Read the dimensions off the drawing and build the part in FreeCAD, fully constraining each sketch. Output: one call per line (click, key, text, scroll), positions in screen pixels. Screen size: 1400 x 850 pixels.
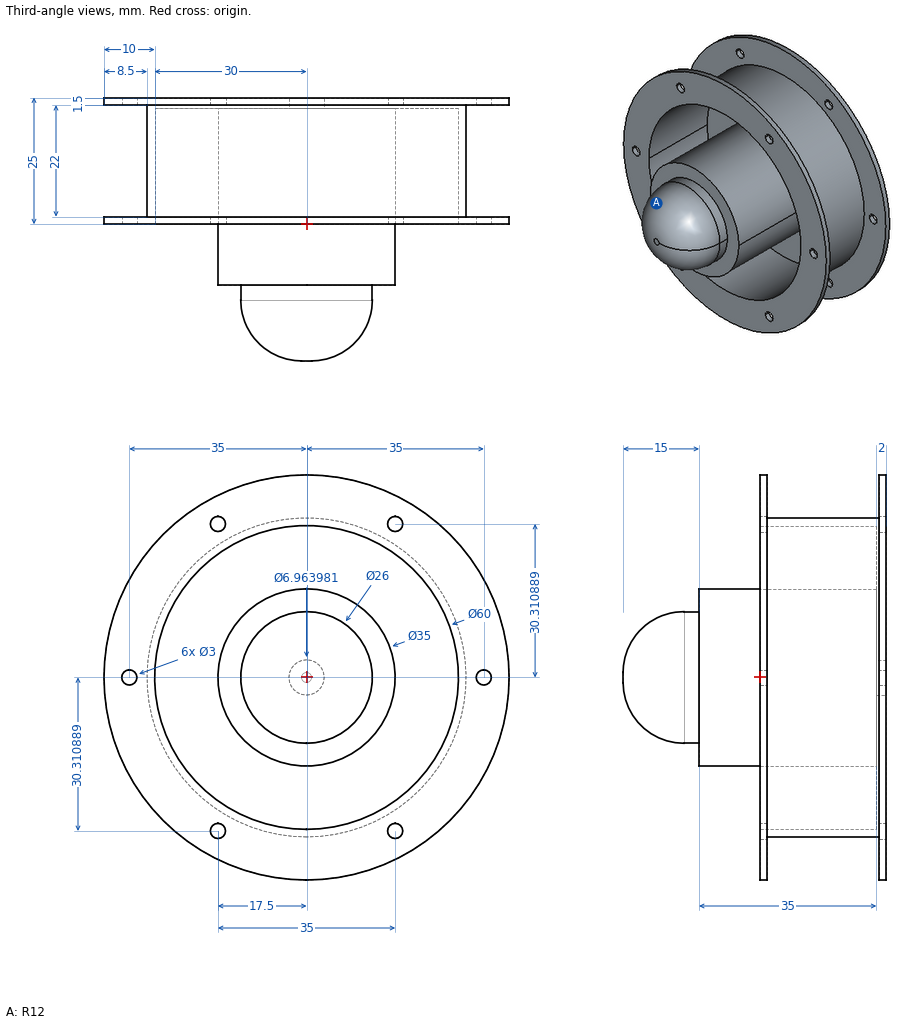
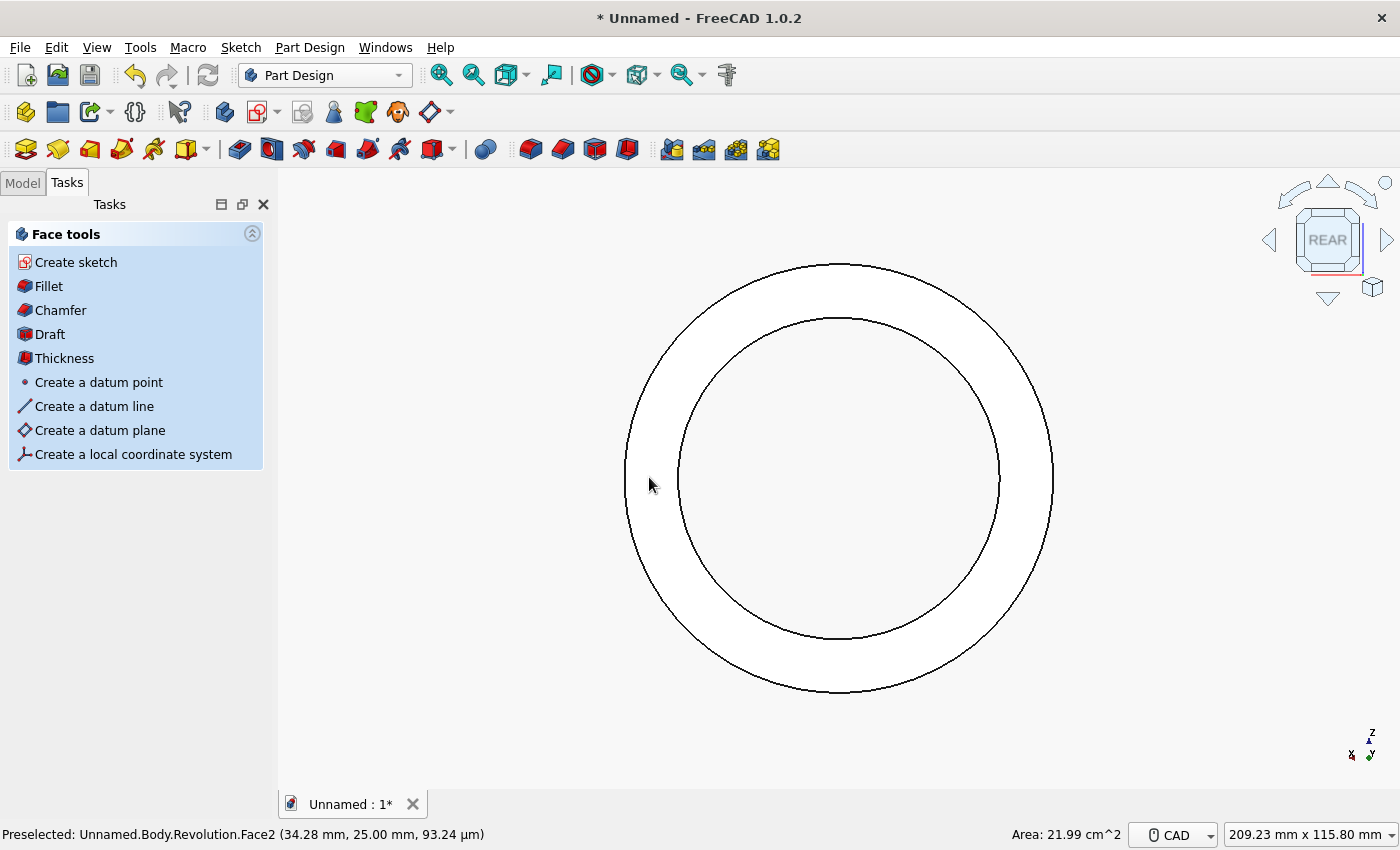
click(258, 112)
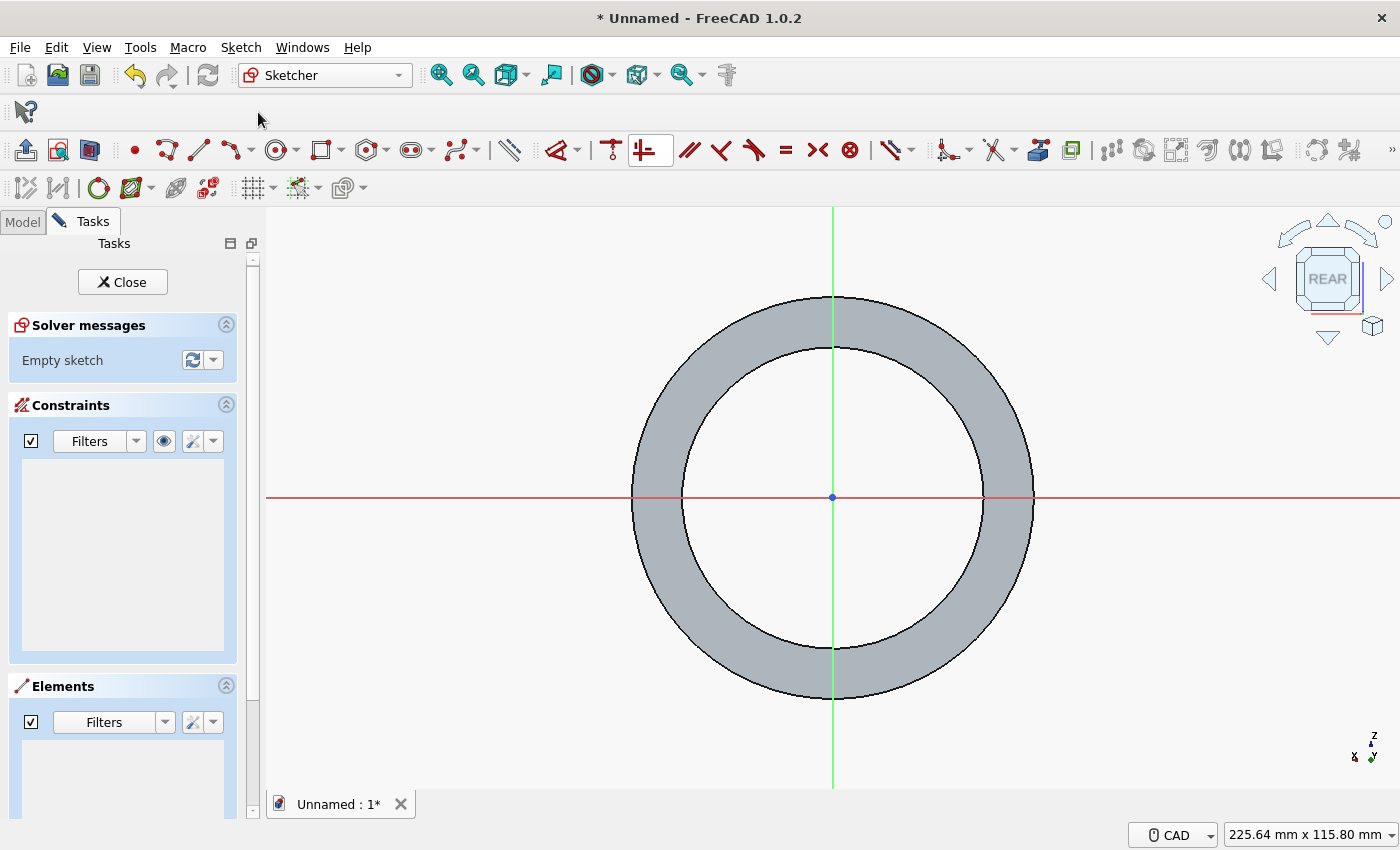
click(276, 150)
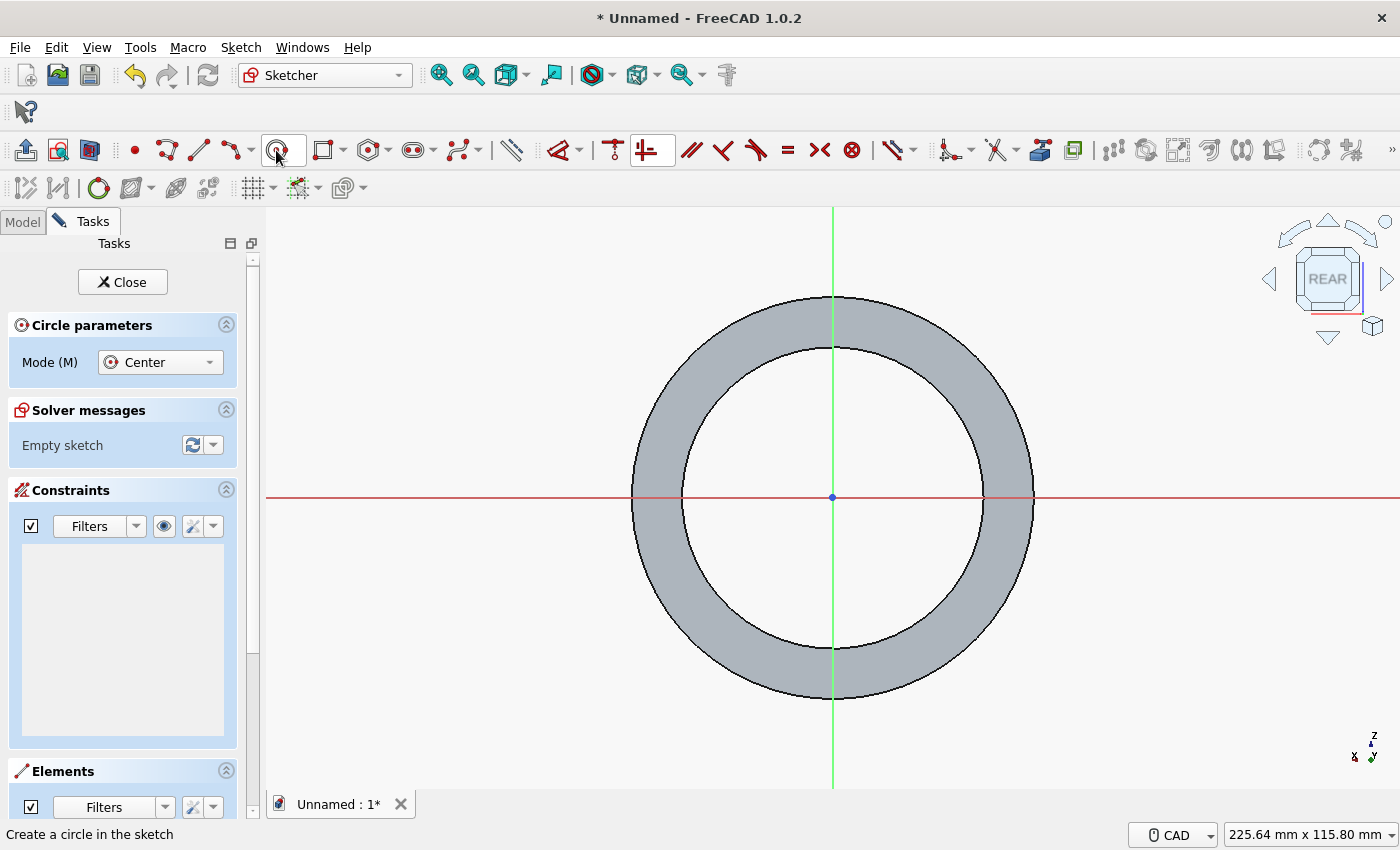
scroll(1009, 498, up, 6)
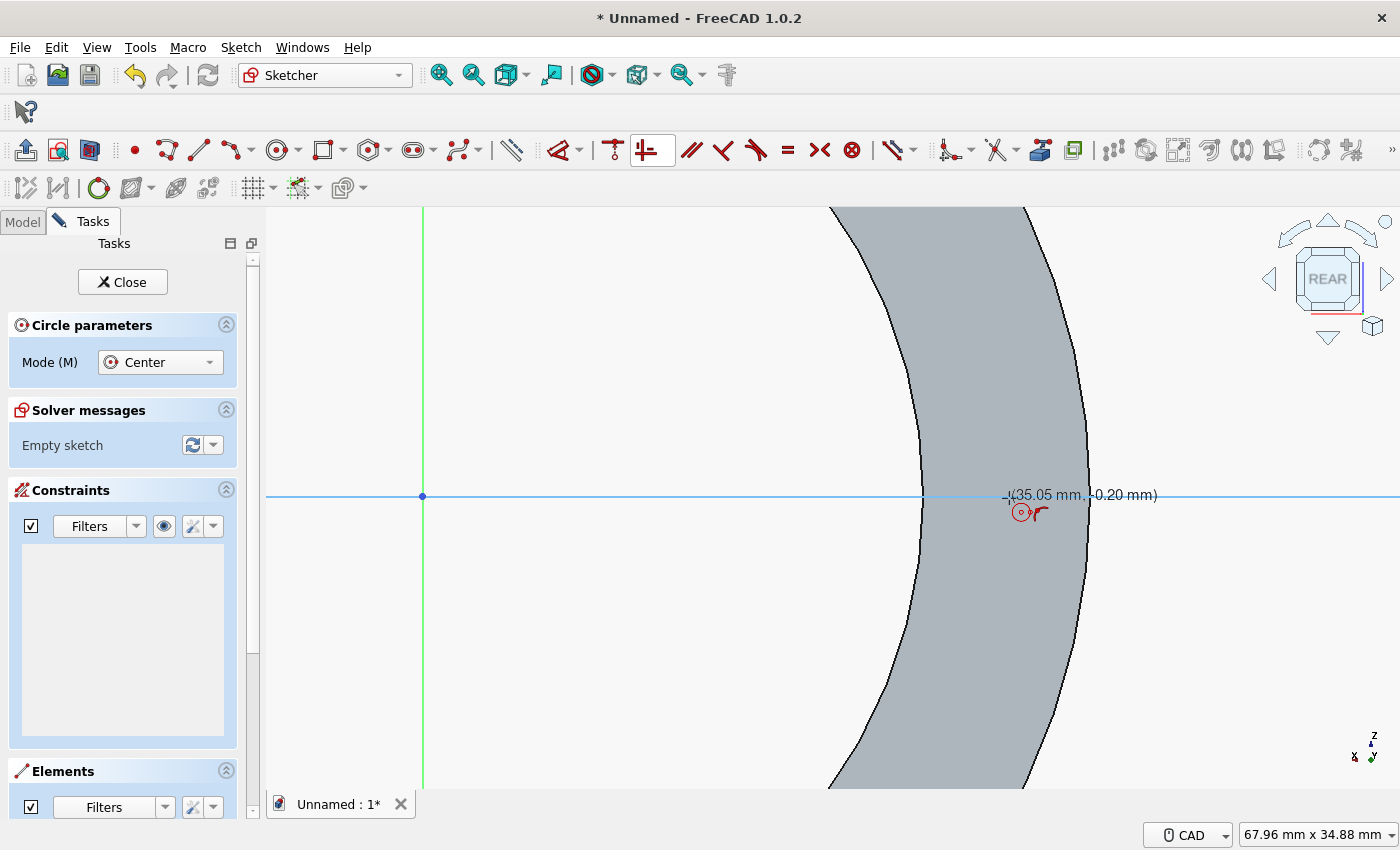
click(1007, 497)
click(1024, 479)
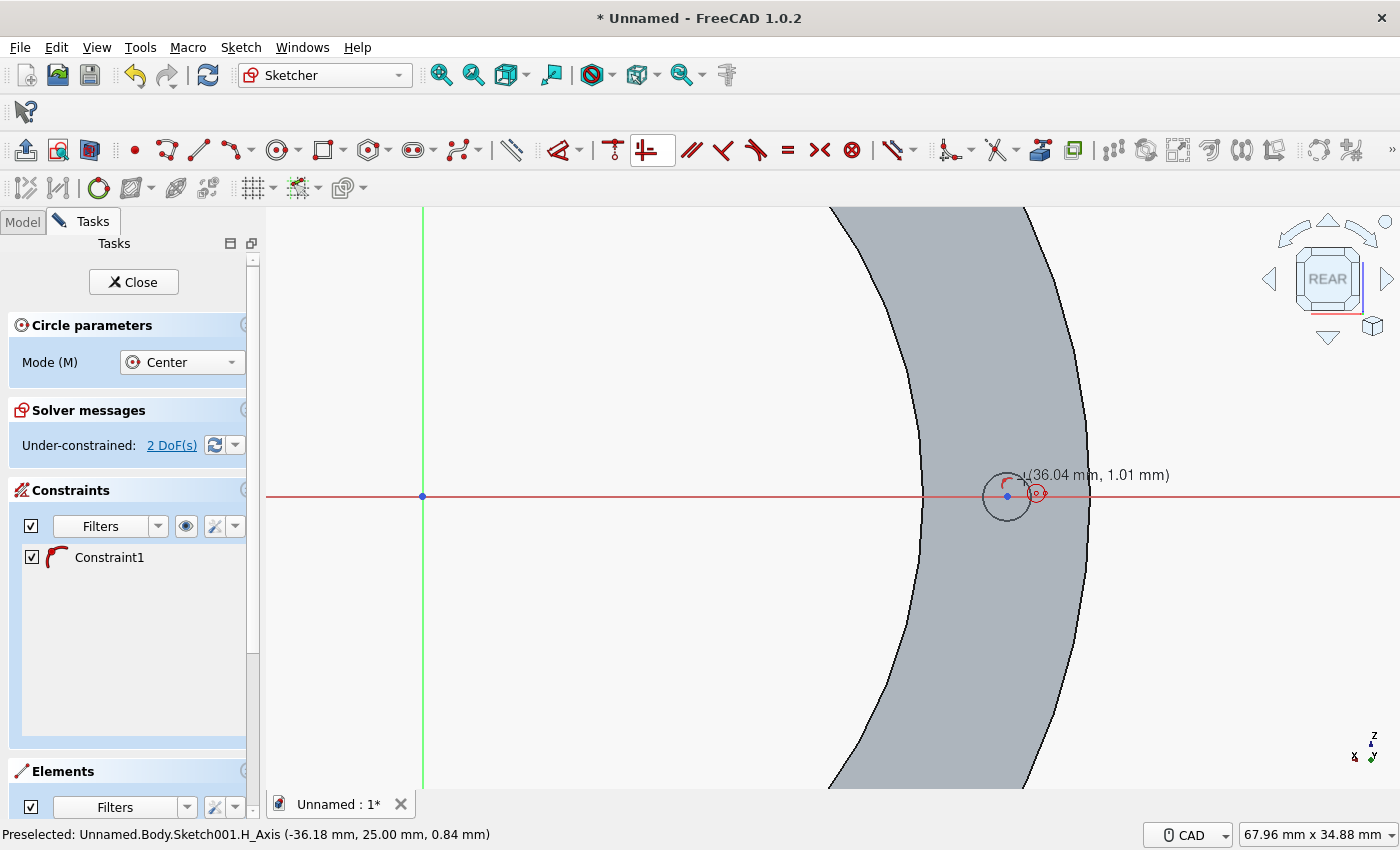
scroll(963, 499, down, 5)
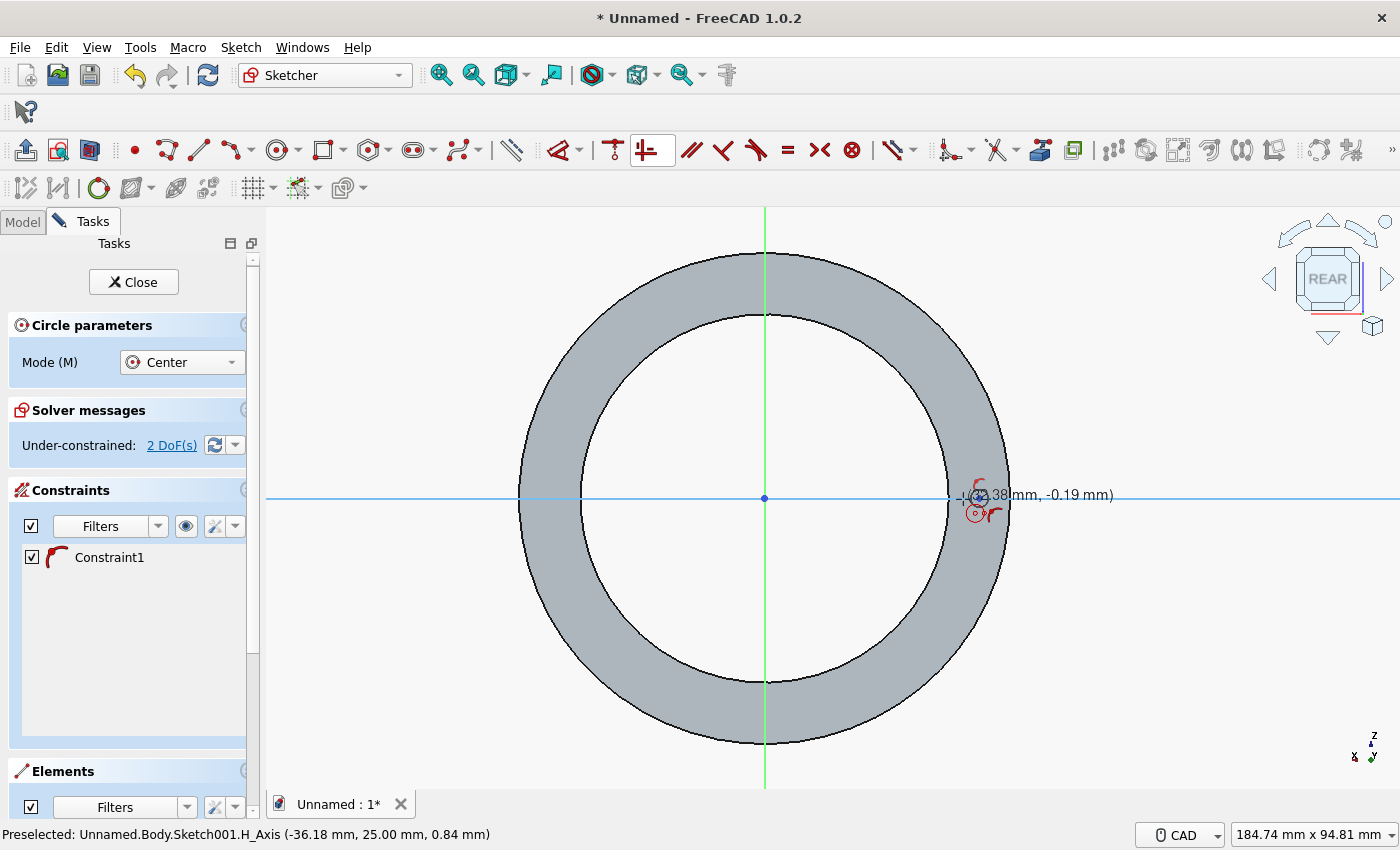
scroll(872, 685, up, 5)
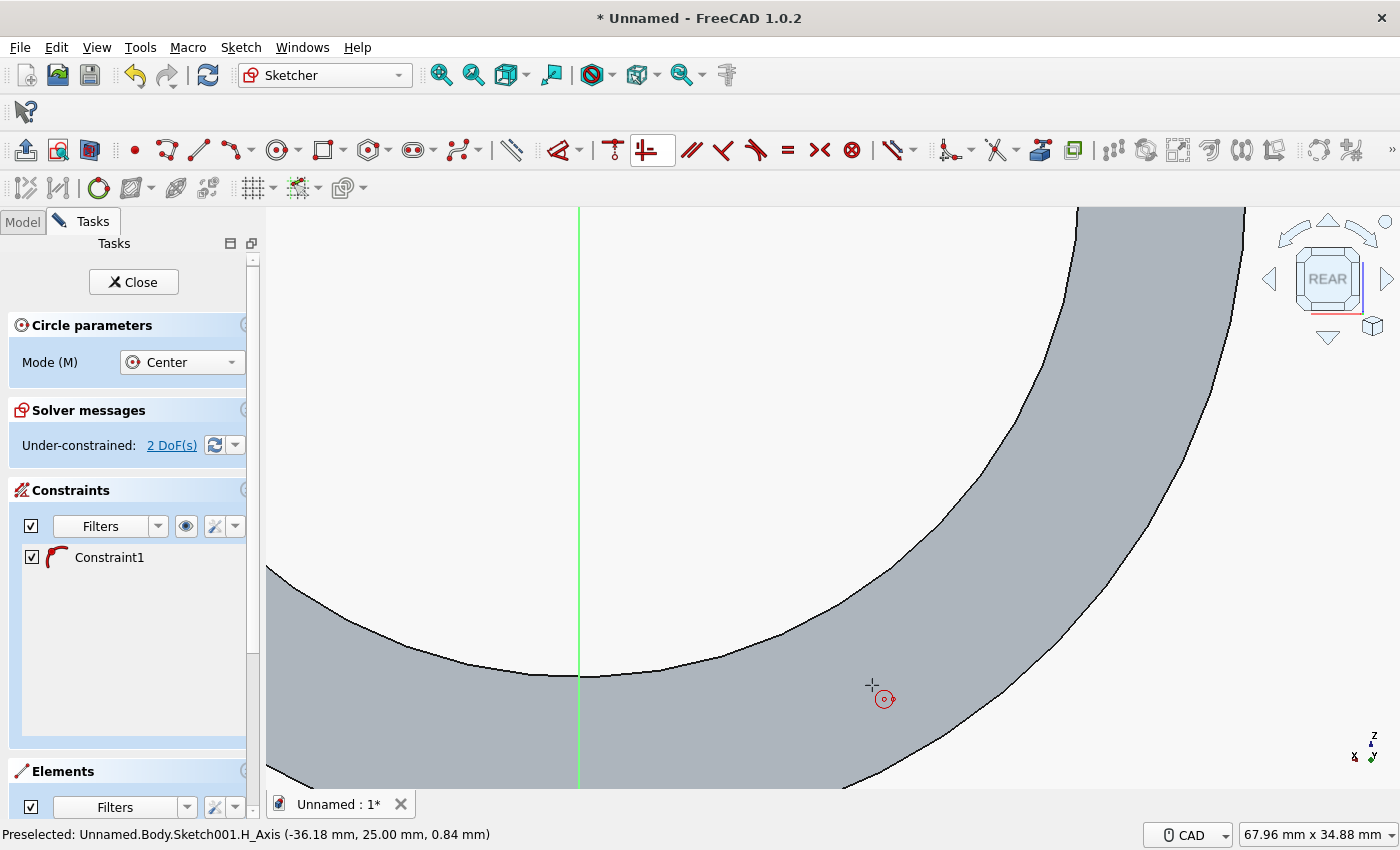
click(871, 682)
click(889, 665)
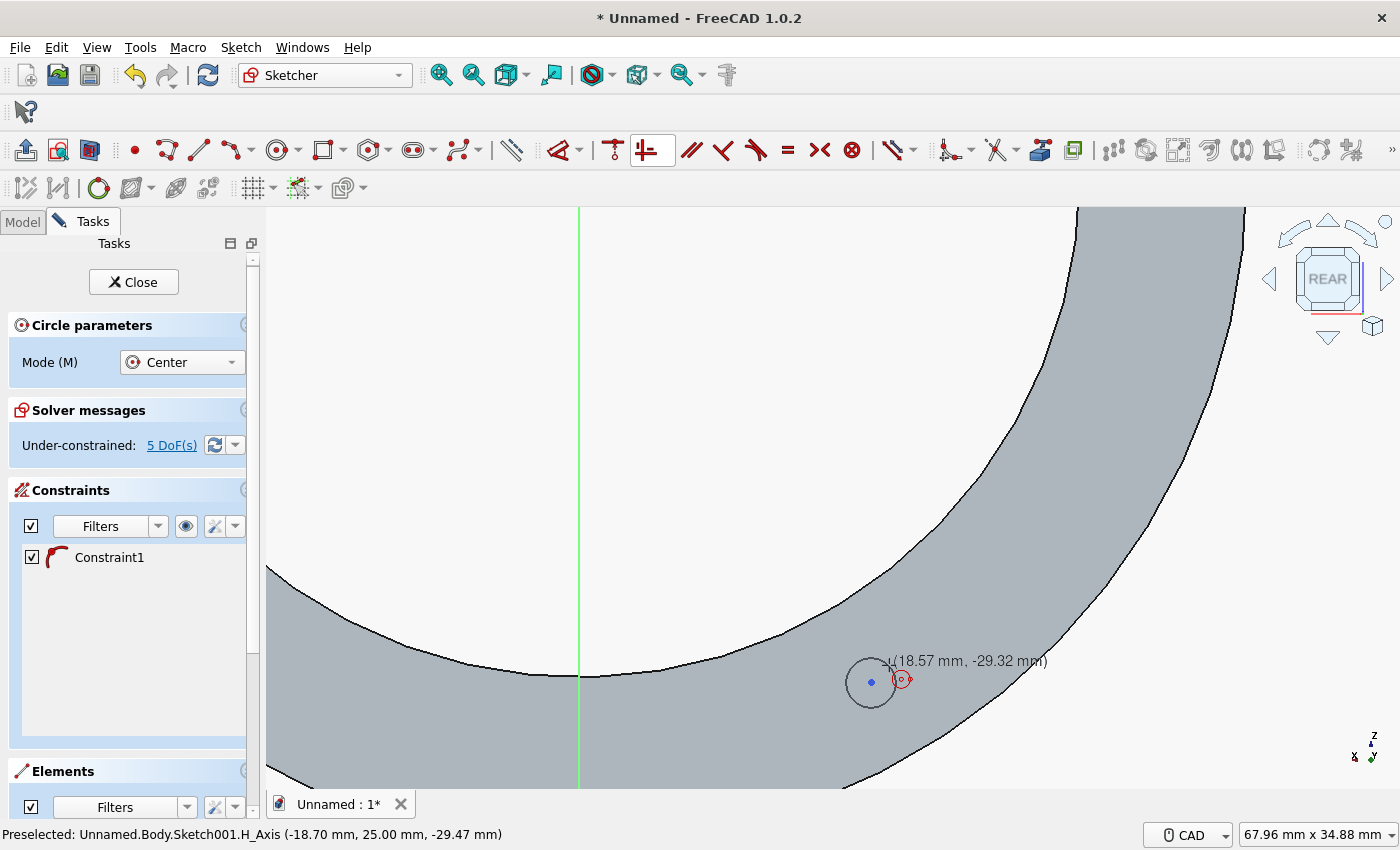
scroll(872, 685, down, 5)